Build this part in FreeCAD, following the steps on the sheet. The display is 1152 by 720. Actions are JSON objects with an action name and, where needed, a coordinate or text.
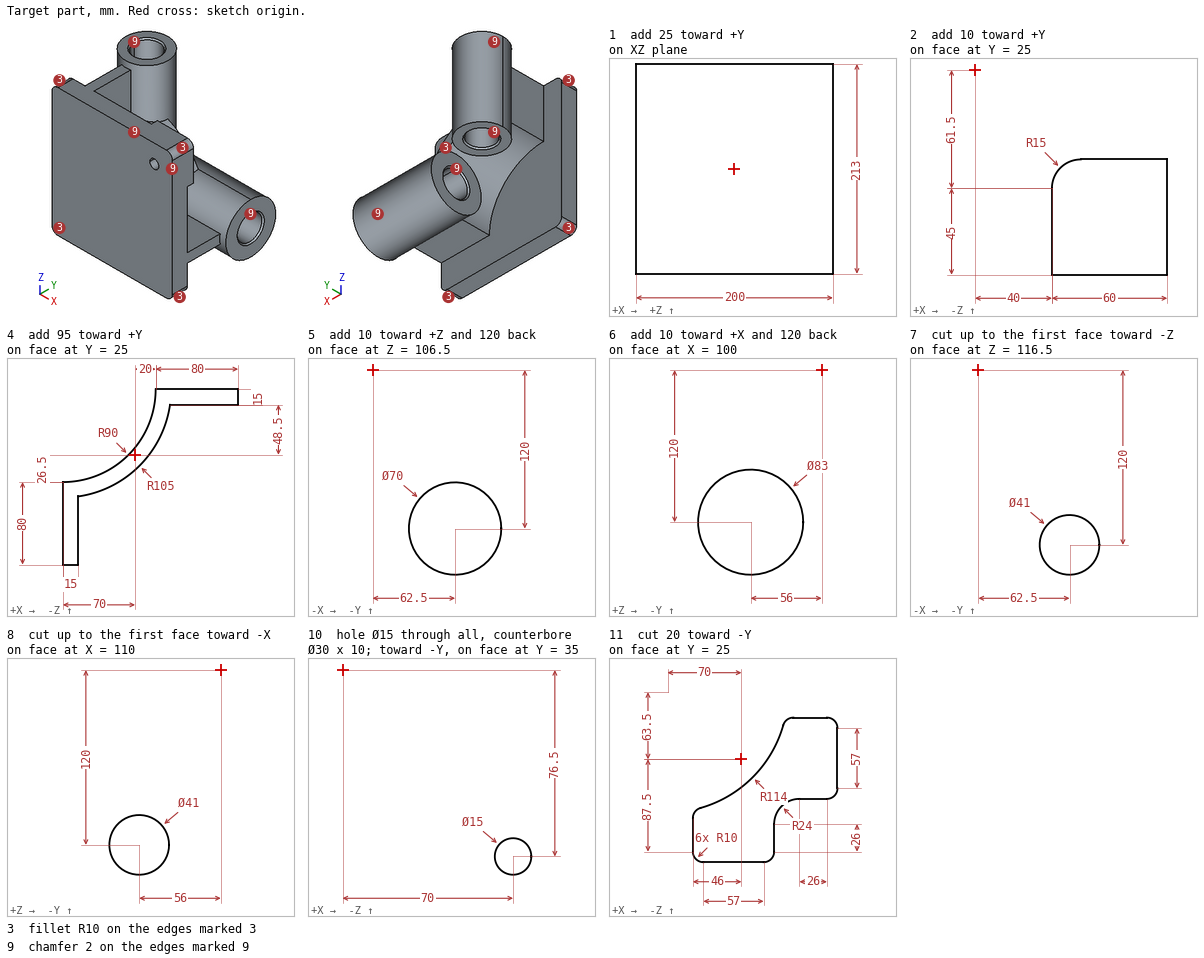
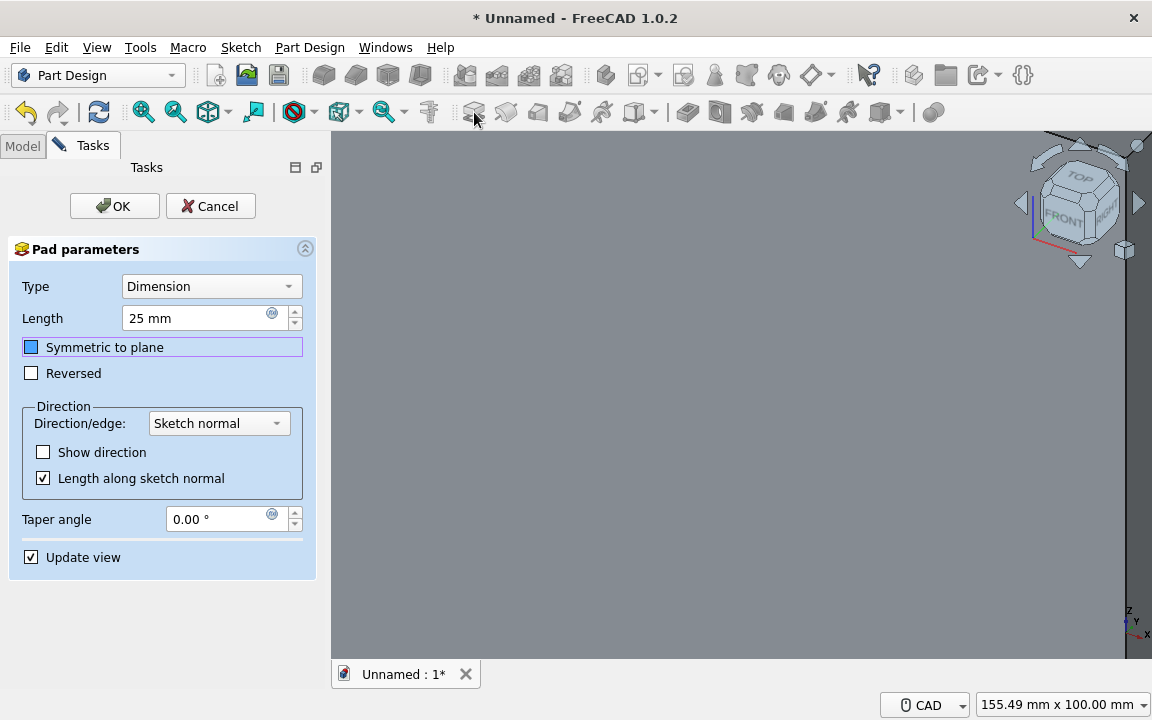
{"action": "left_click", "coordinate": [30, 373]}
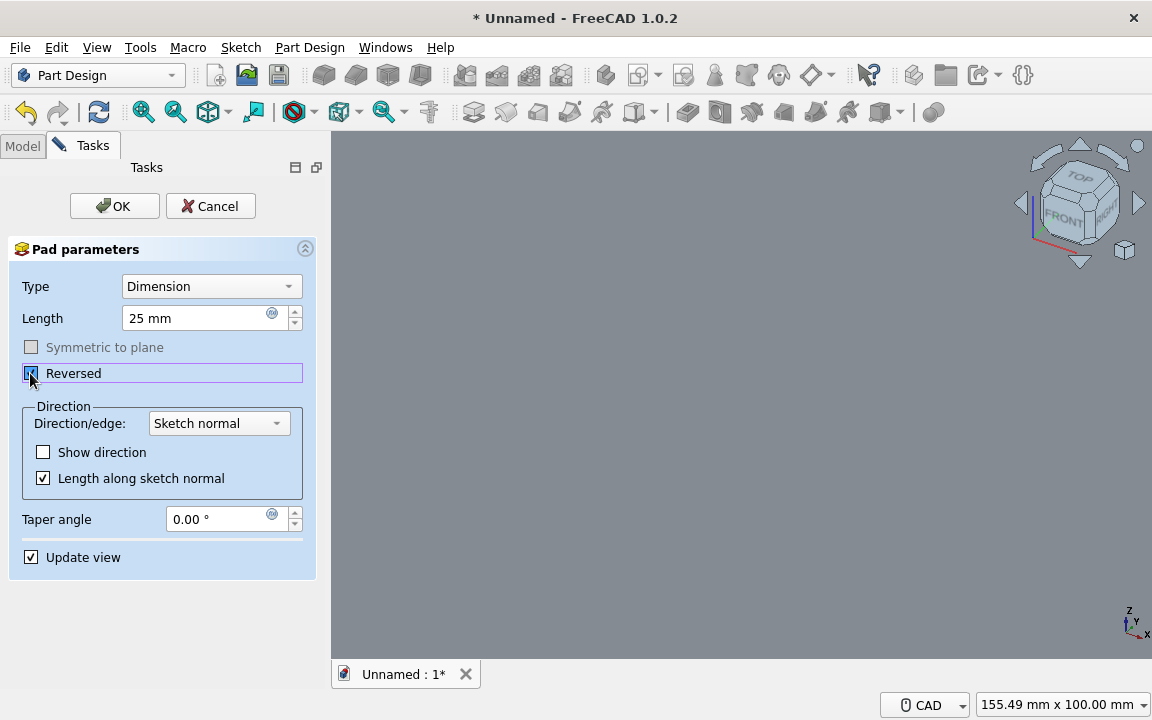
{"action": "left_click", "coordinate": [115, 206]}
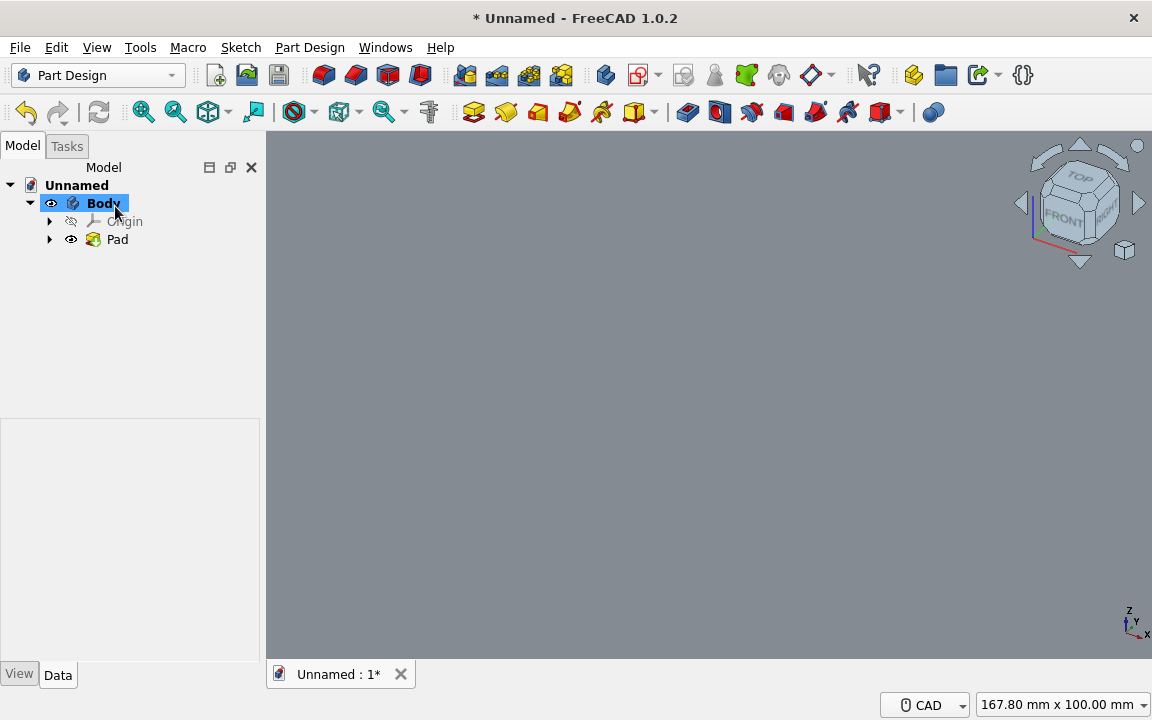
{"action": "left_click", "coordinate": [144, 112]}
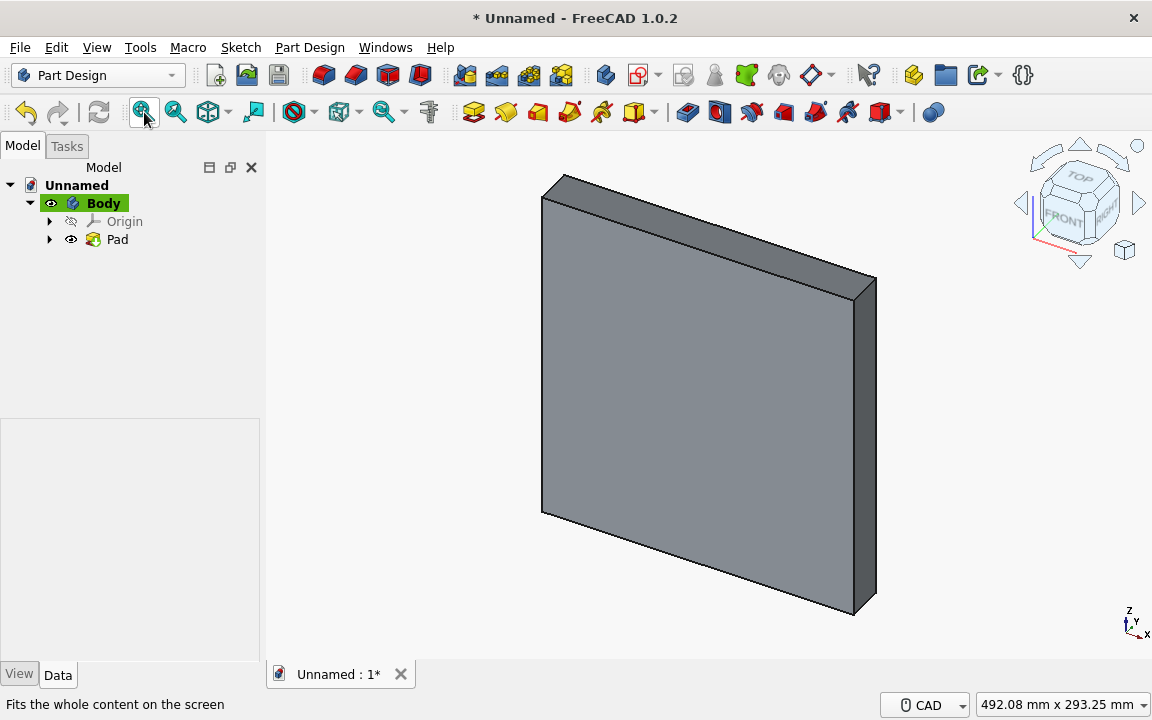
{"action": "key", "text": "4"}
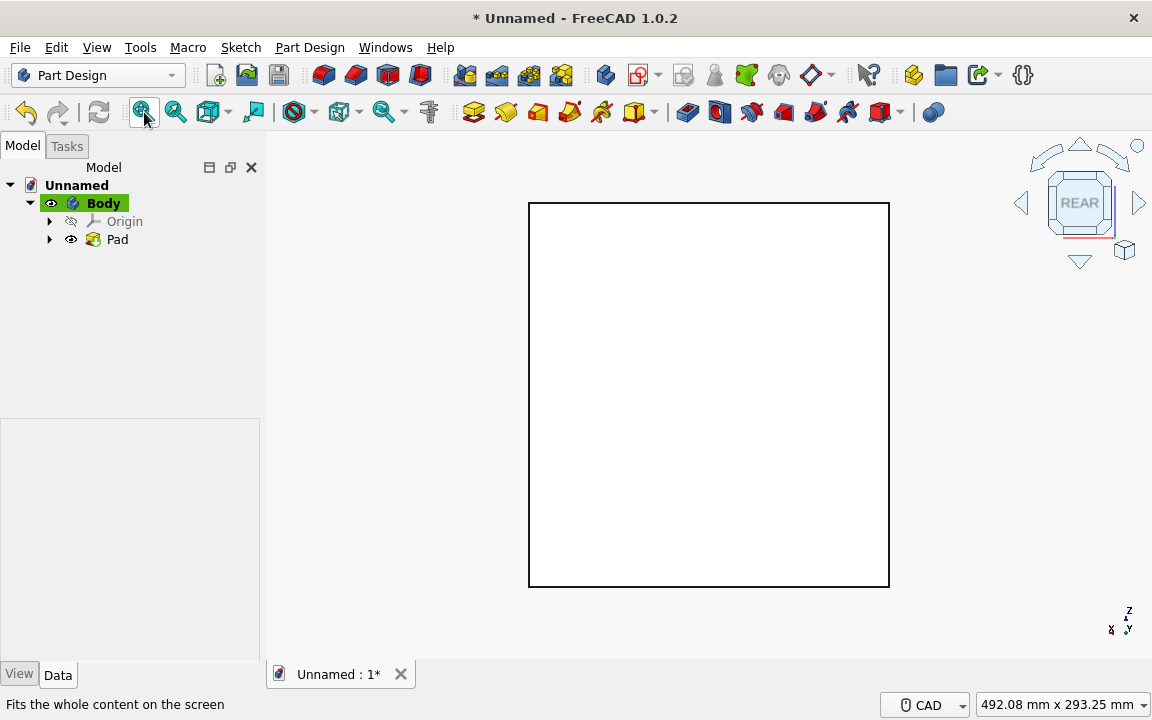
{"action": "left_click", "coordinate": [709, 394]}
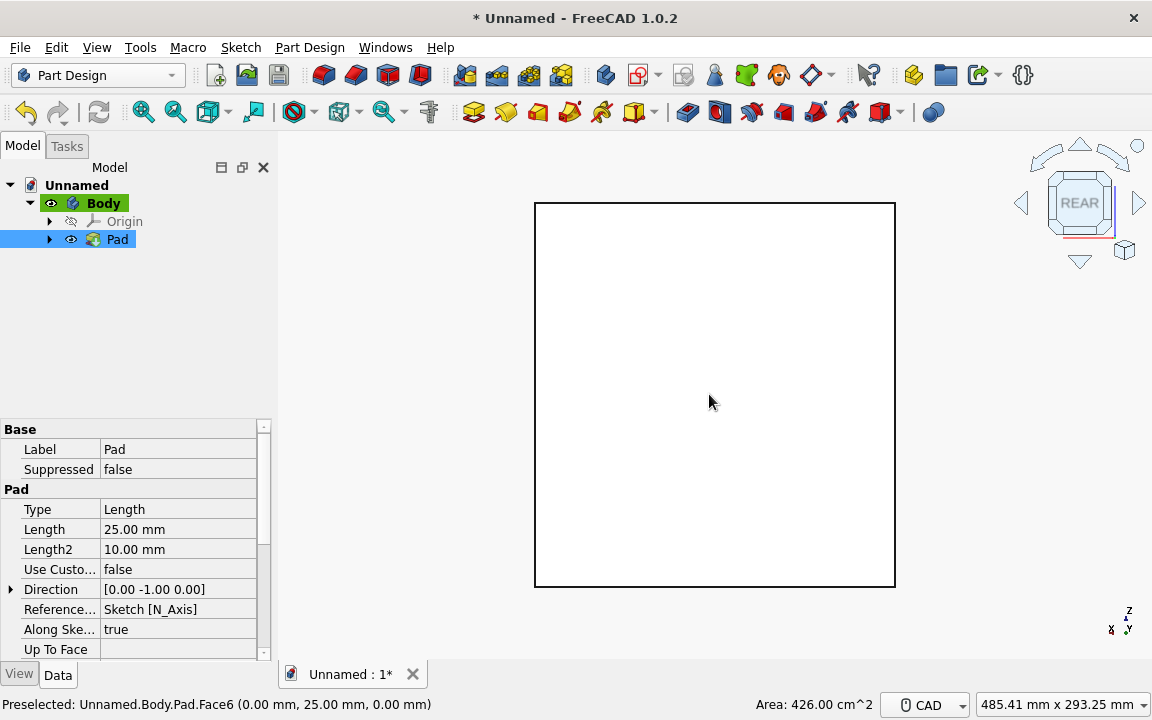
{"action": "left_click", "coordinate": [638, 76]}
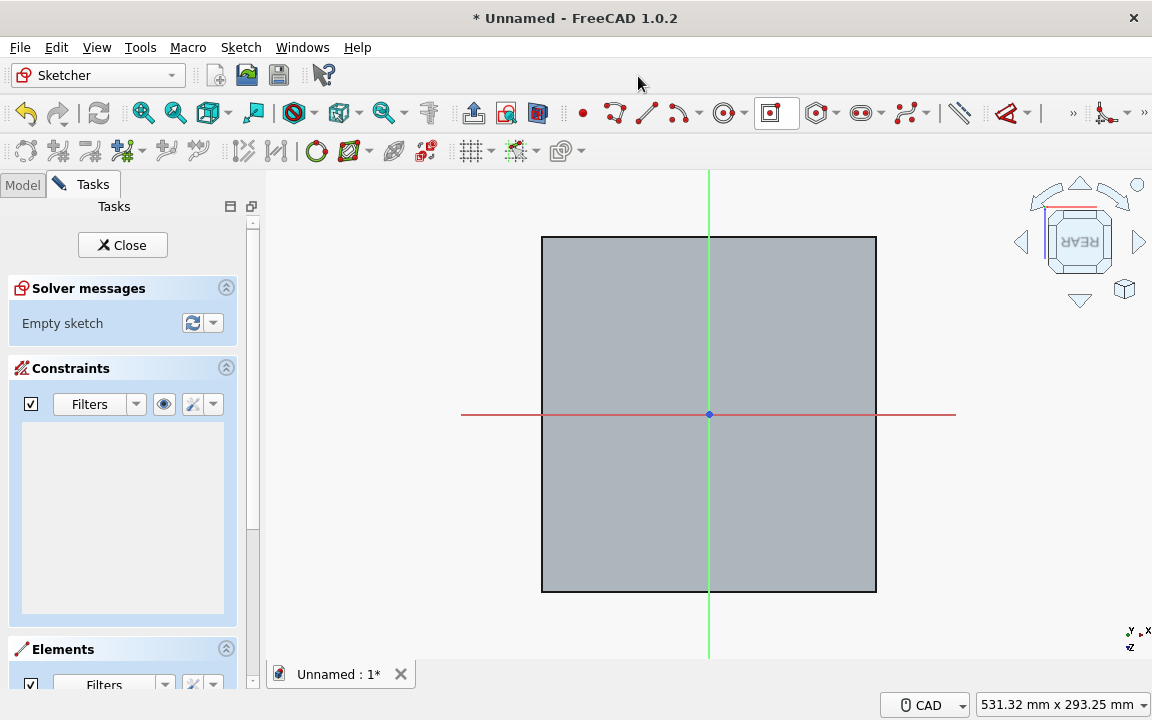
{"action": "scroll", "coordinate": [977, 611], "scroll_direction": "up", "scroll_amount": 3}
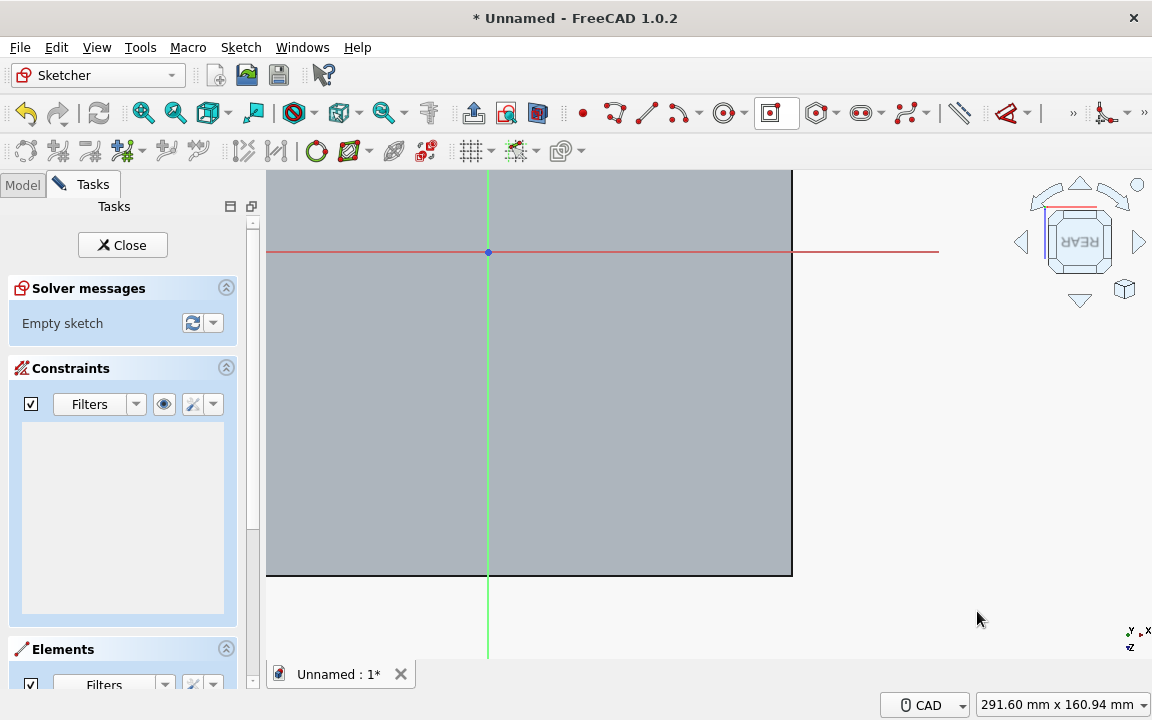
{"action": "left_click", "coordinate": [616, 114]}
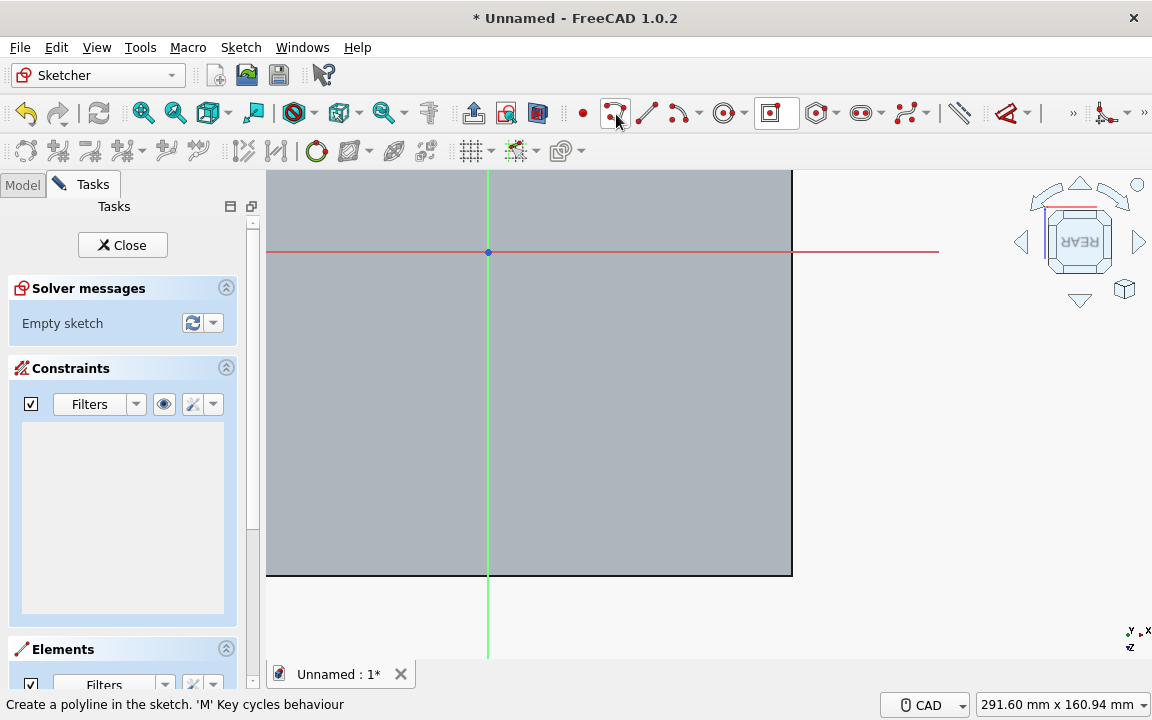
{"action": "left_click", "coordinate": [610, 439]}
{"action": "left_click", "coordinate": [610, 576]}
{"action": "left_click", "coordinate": [792, 576]}
{"action": "left_click", "coordinate": [792, 393]}
{"action": "left_click", "coordinate": [655, 393]}
{"action": "right_click", "coordinate": [655, 393]}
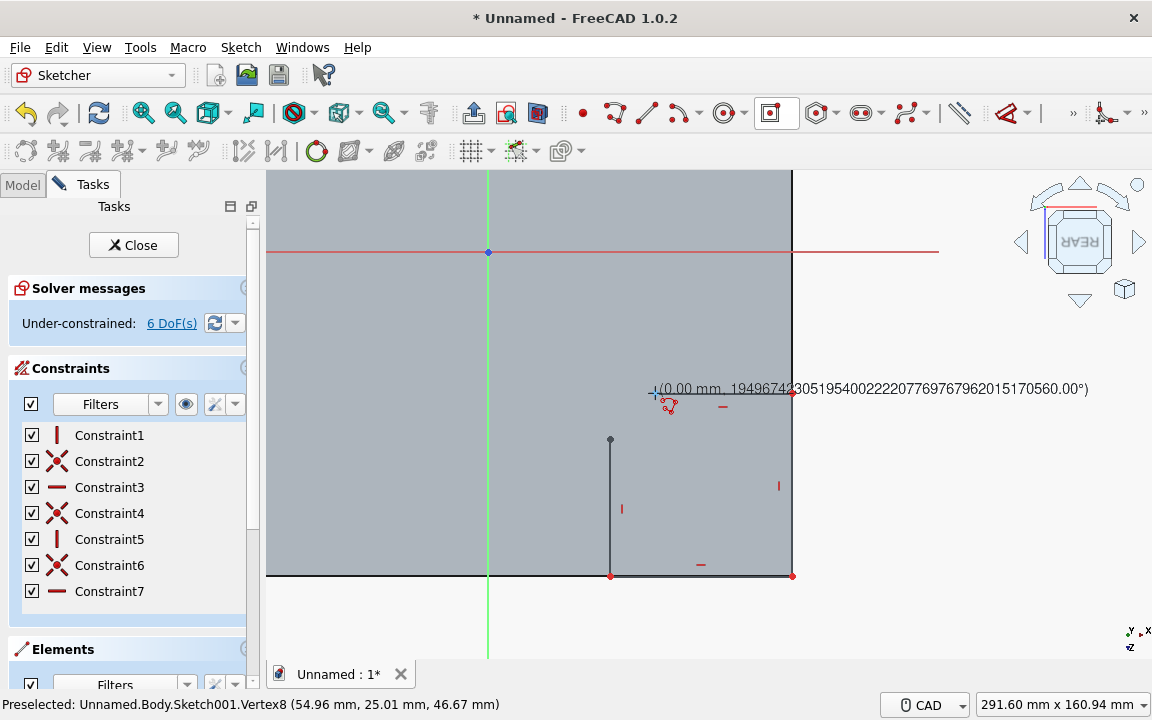
{"action": "key", "text": "g 3 a"}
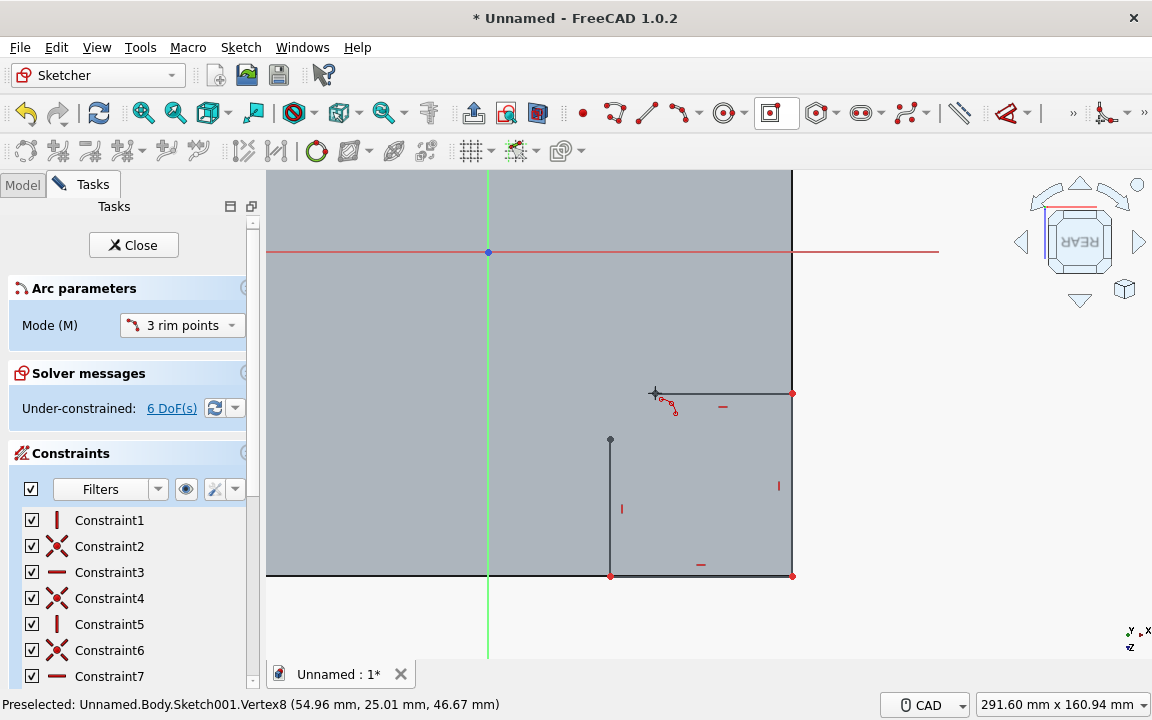
{"action": "left_click", "coordinate": [655, 394]}
{"action": "left_click", "coordinate": [610, 440]}
{"action": "left_click", "coordinate": [623, 407]}
{"action": "key", "text": "Escape"}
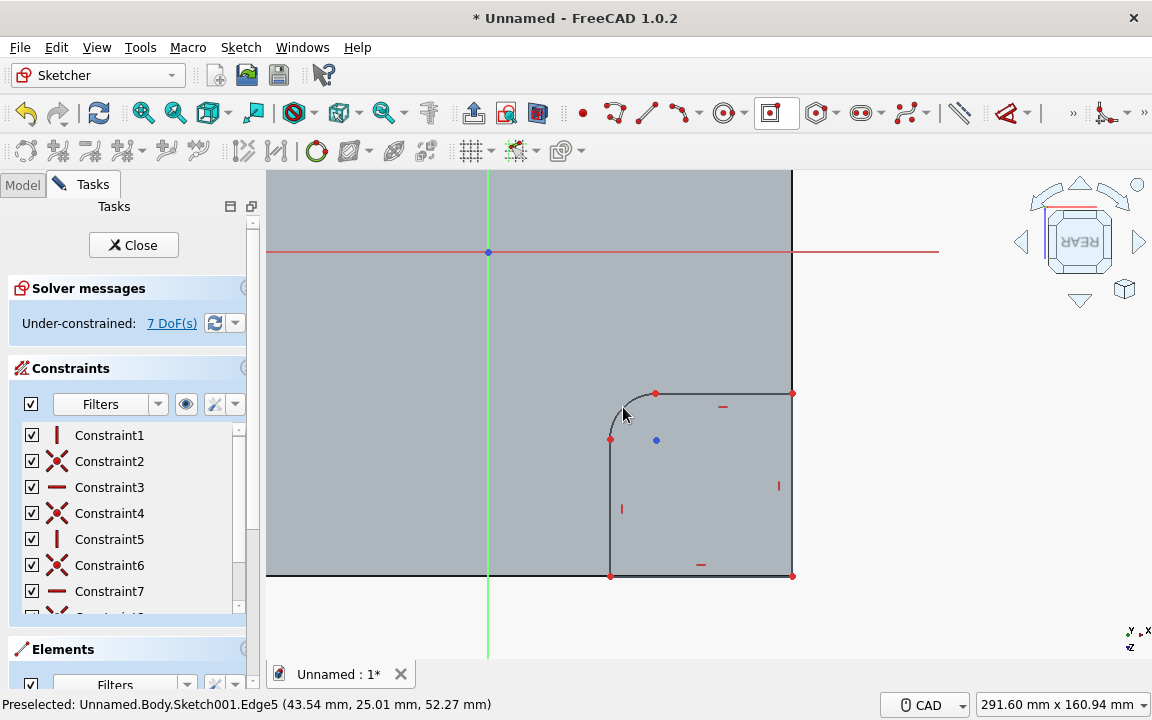
{"action": "left_click", "coordinate": [610, 481]}